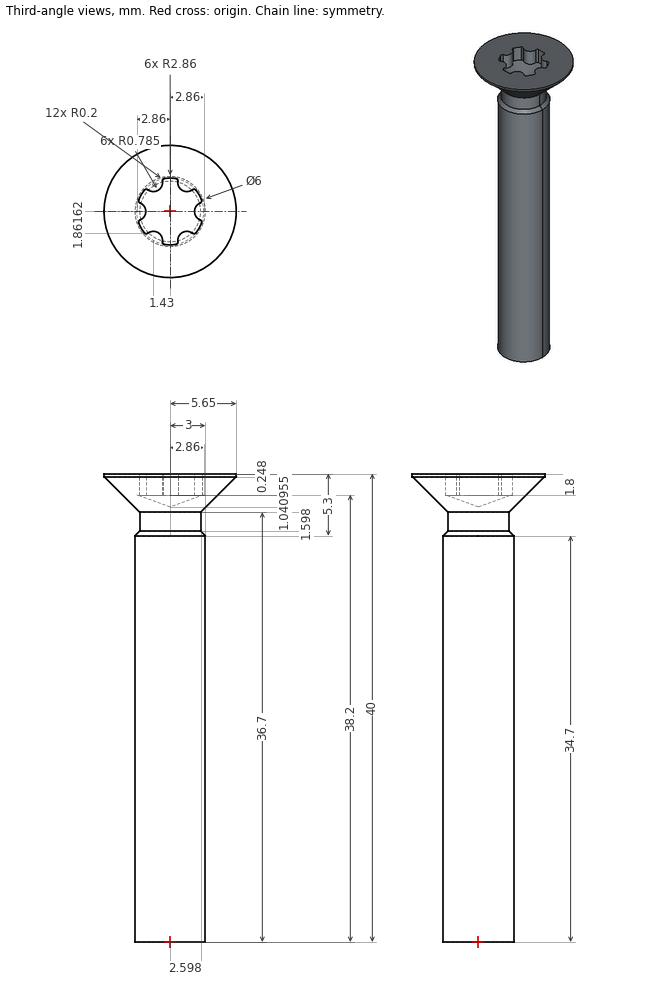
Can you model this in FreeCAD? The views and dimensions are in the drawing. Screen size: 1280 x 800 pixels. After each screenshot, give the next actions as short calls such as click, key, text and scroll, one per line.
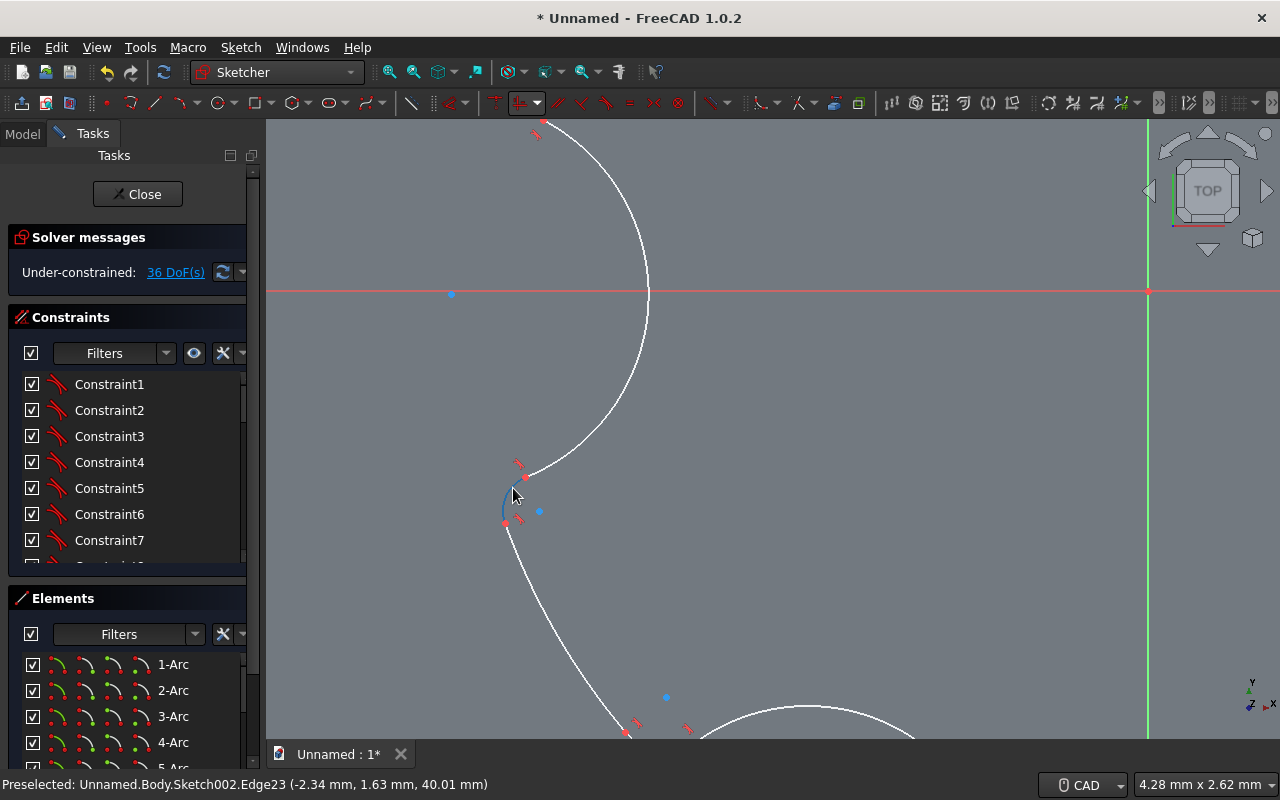
click(512, 487)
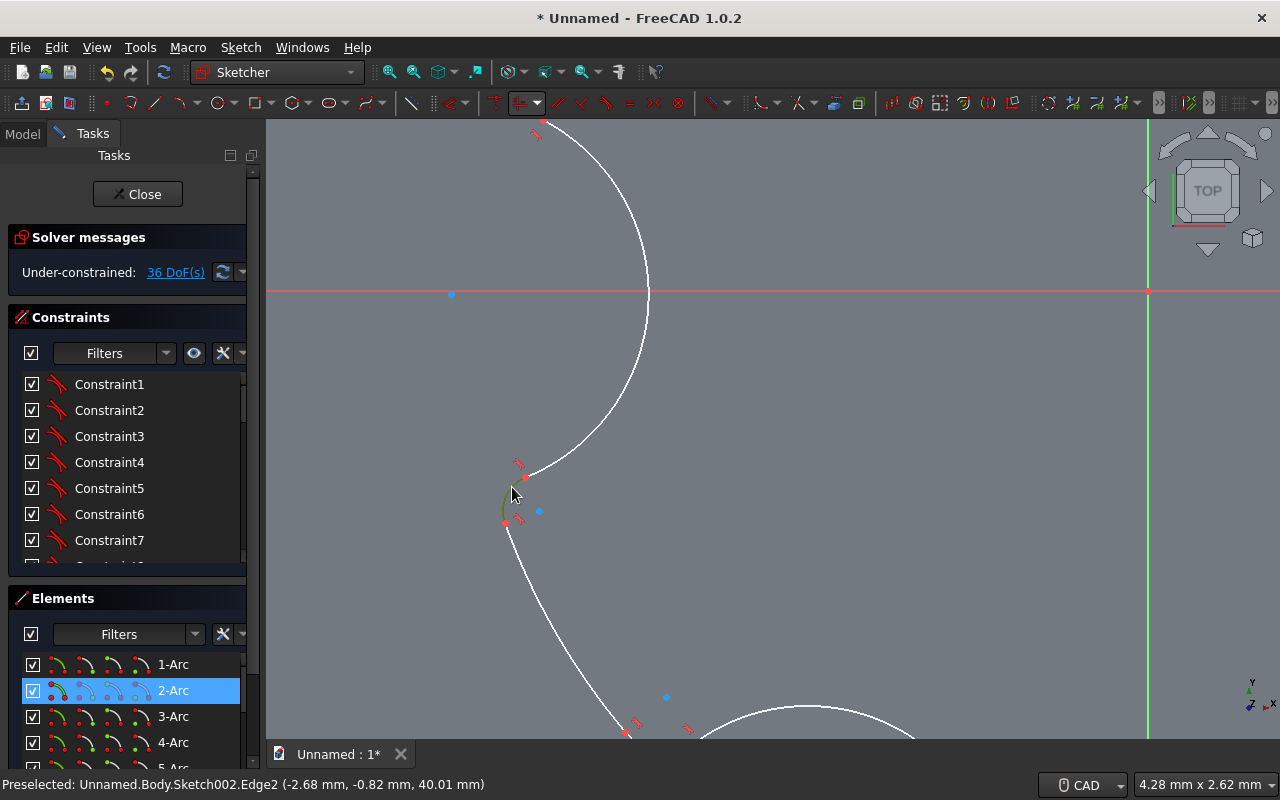
scroll(513, 488, down, 6)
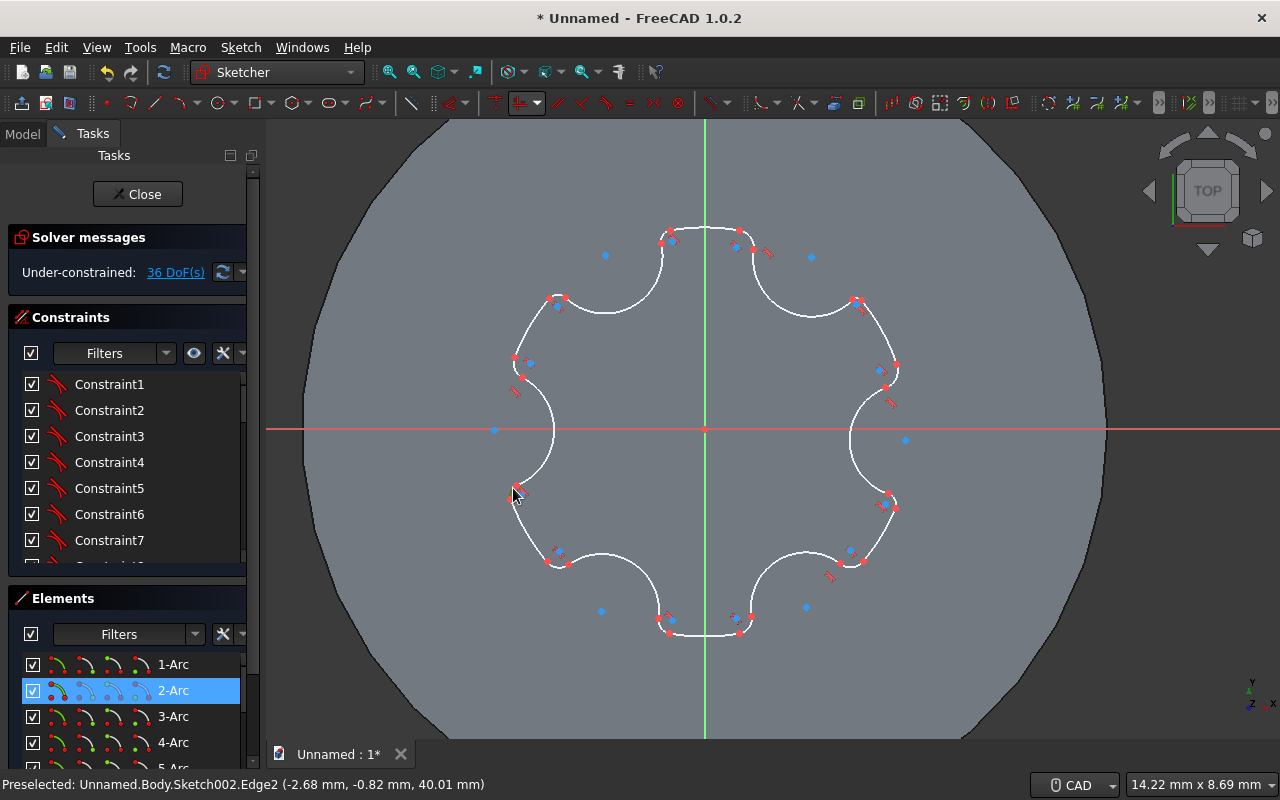
scroll(553, 566, up, 4)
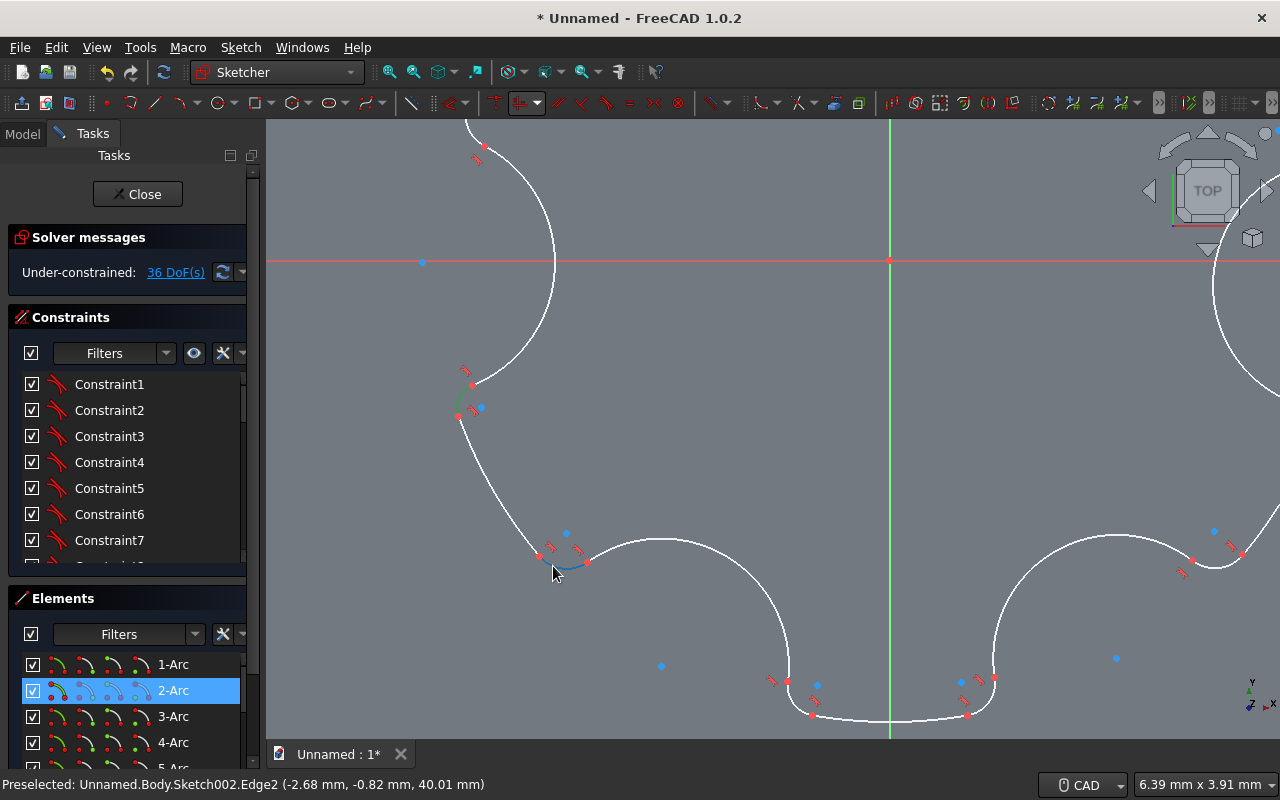
click(552, 566)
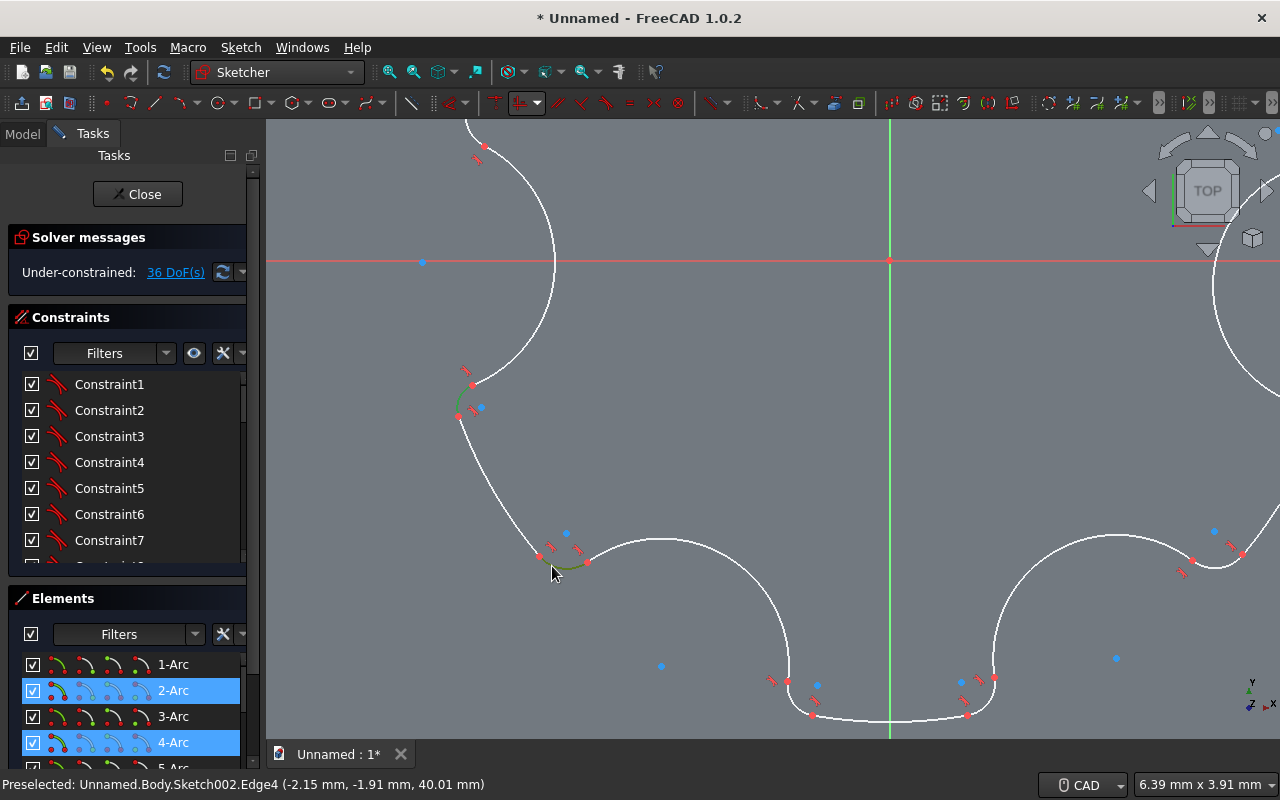
click(789, 696)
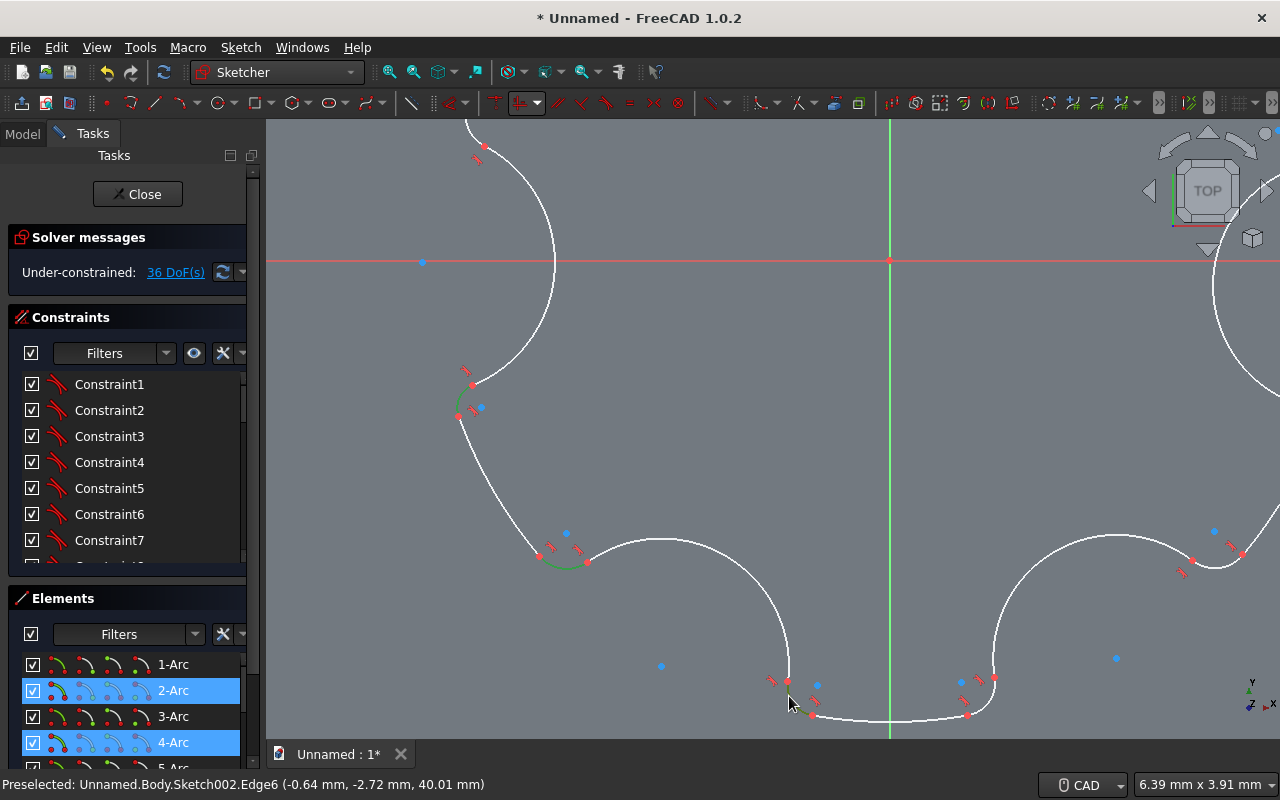
click(982, 709)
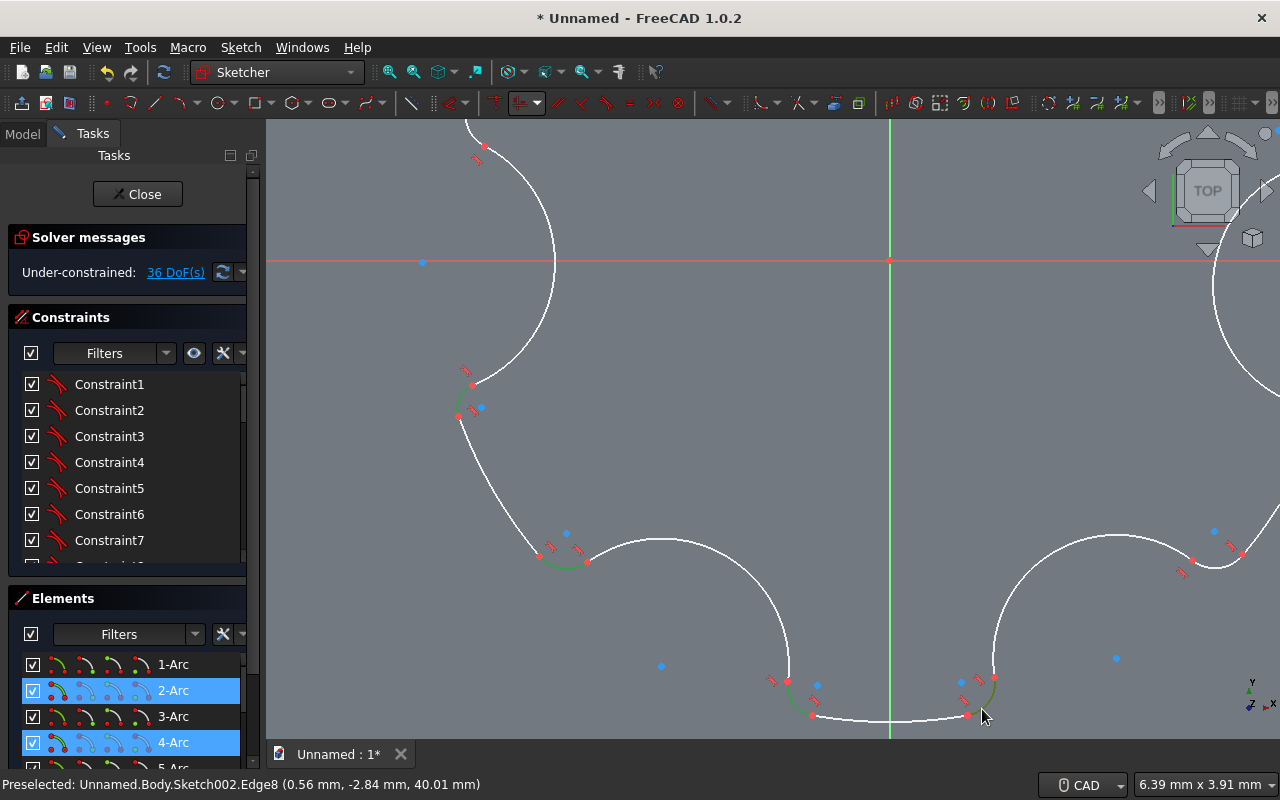
scroll(553, 566, down, 4)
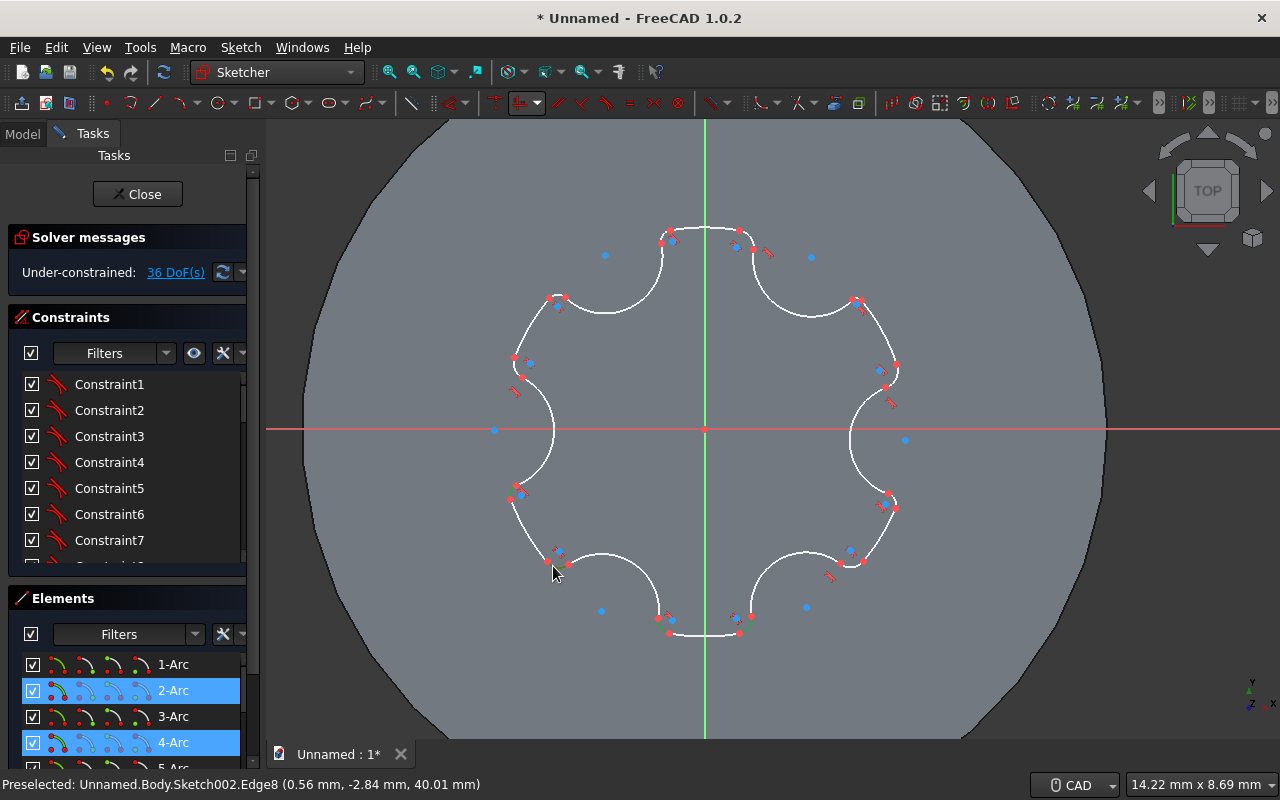
scroll(847, 567, up, 4)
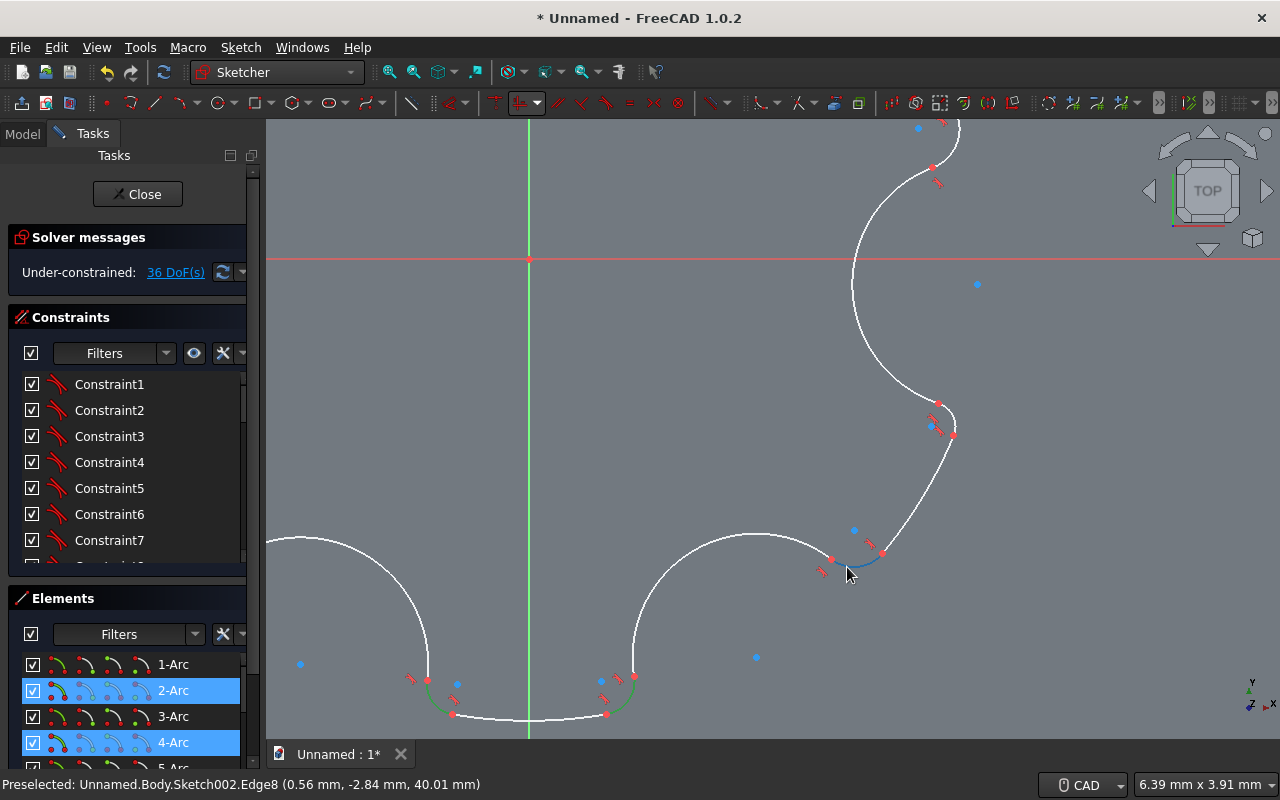
click(847, 566)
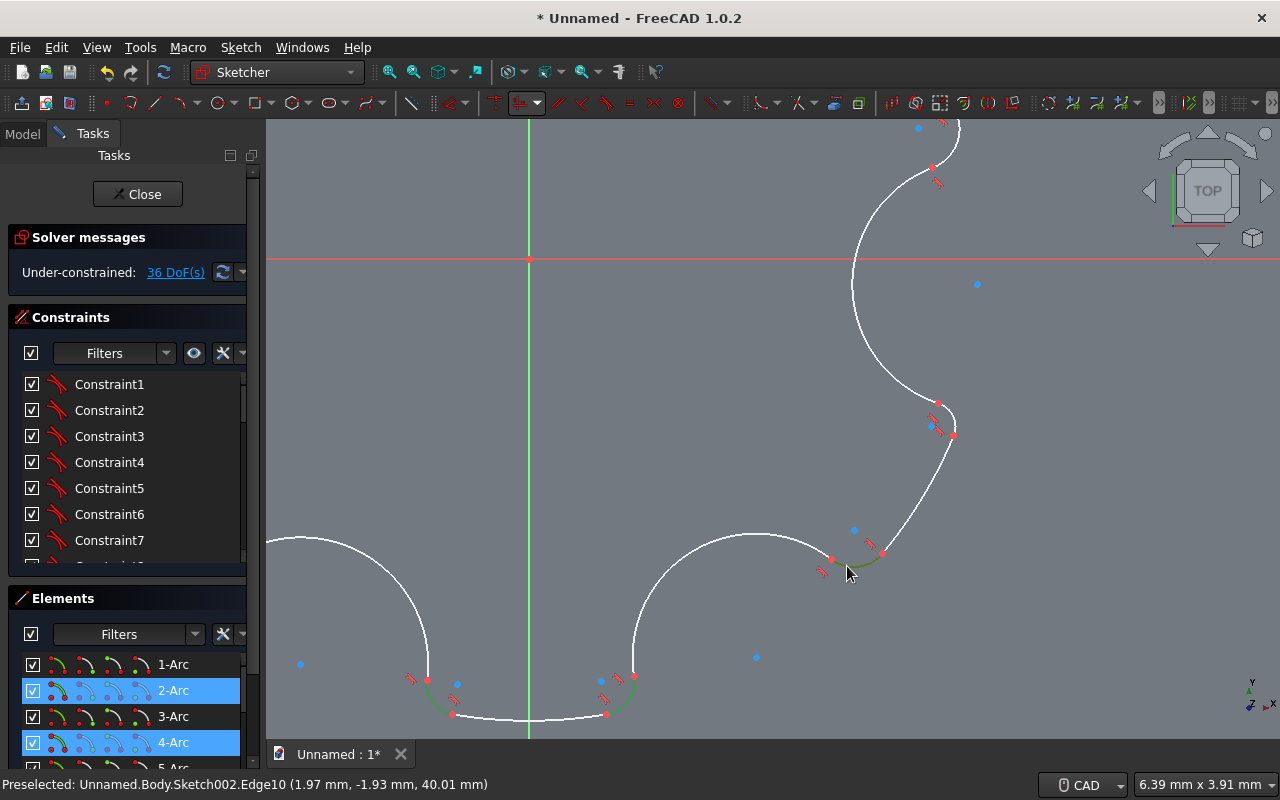
click(955, 424)